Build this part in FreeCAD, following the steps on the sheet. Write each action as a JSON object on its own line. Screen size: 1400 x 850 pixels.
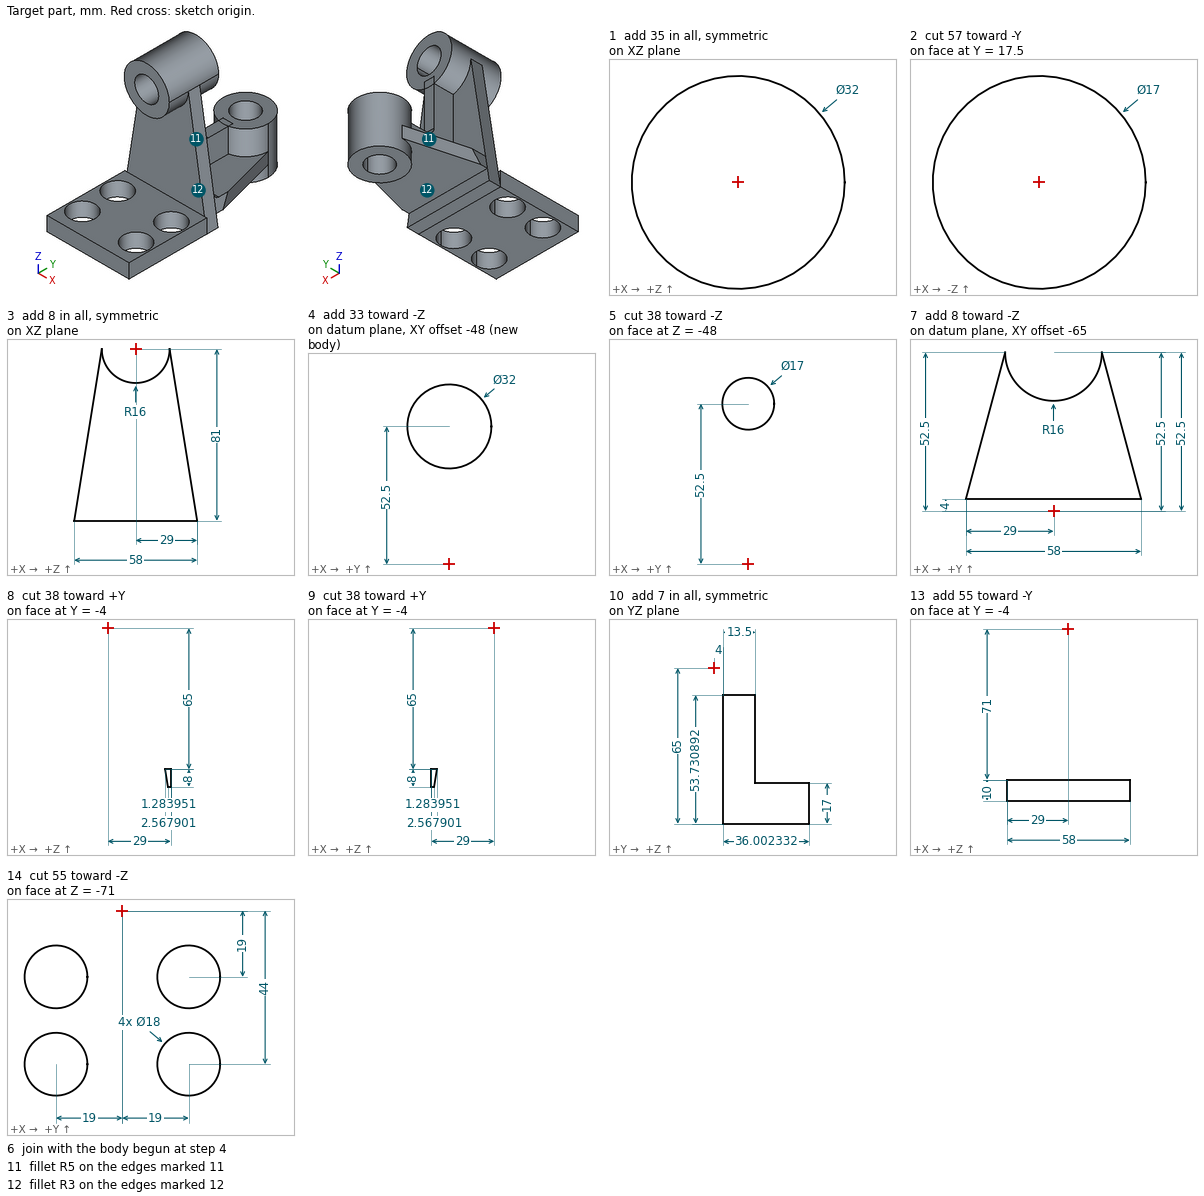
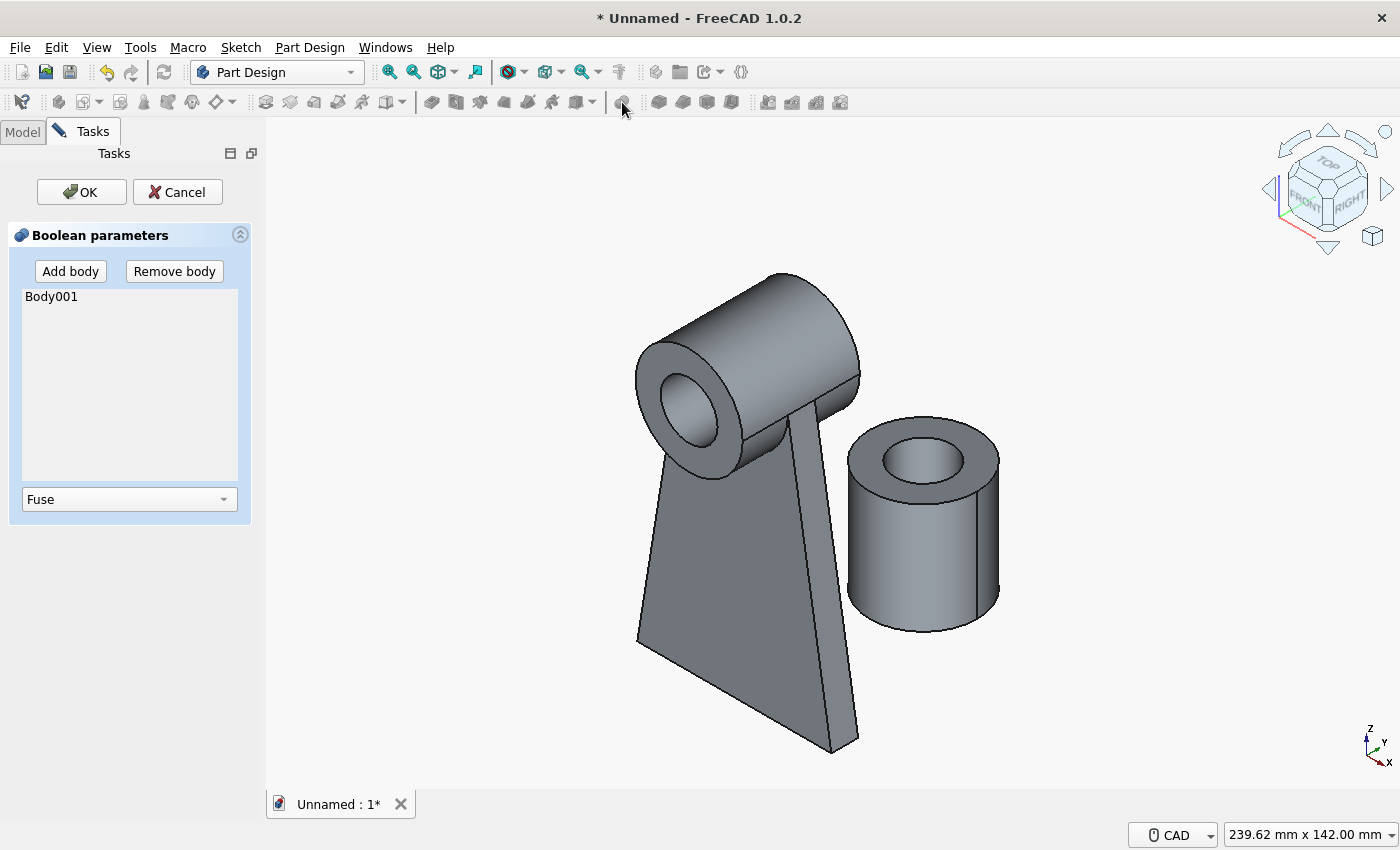
{"action": "left_click", "coordinate": [82, 192]}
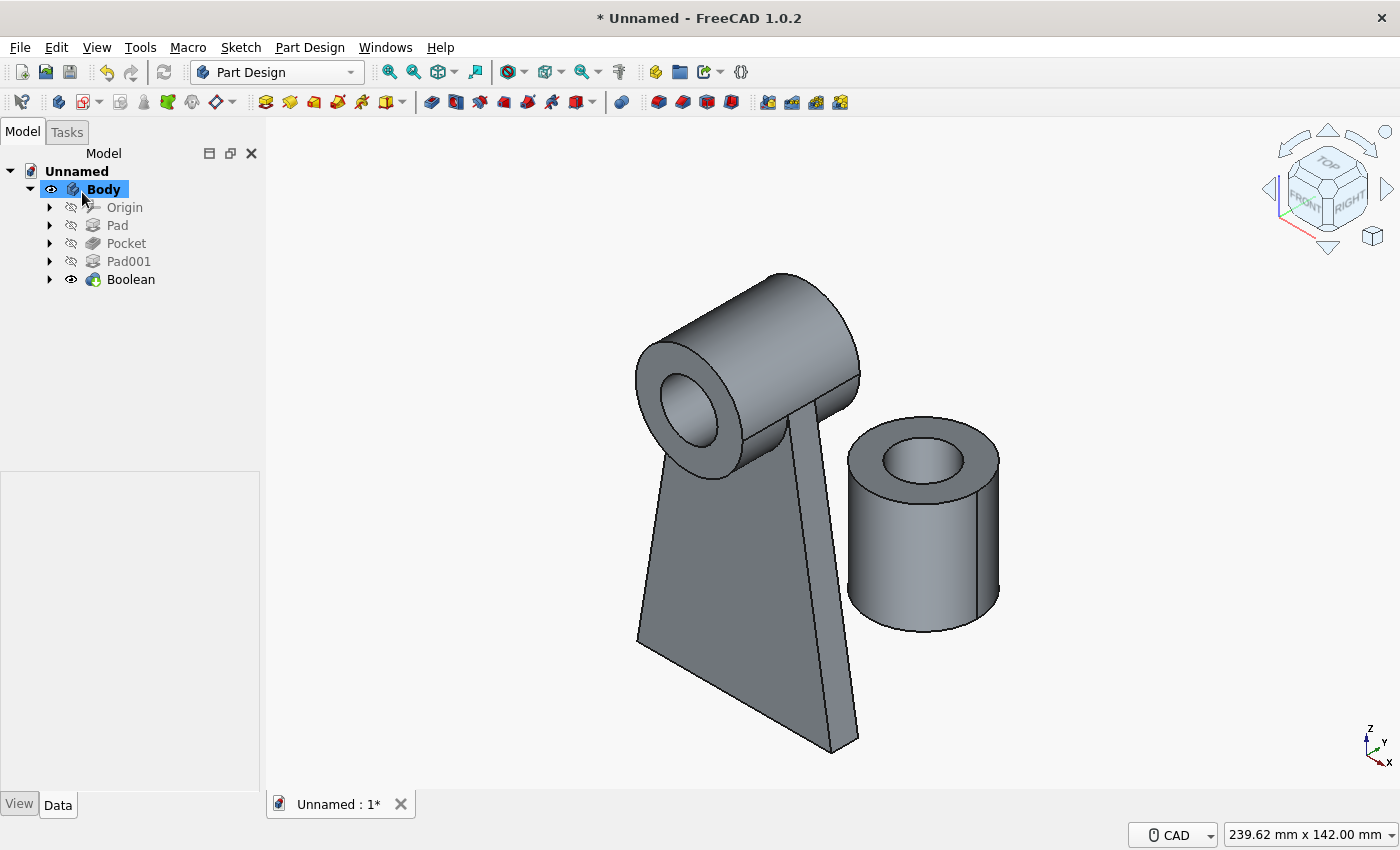
{"action": "left_click", "coordinate": [50, 207]}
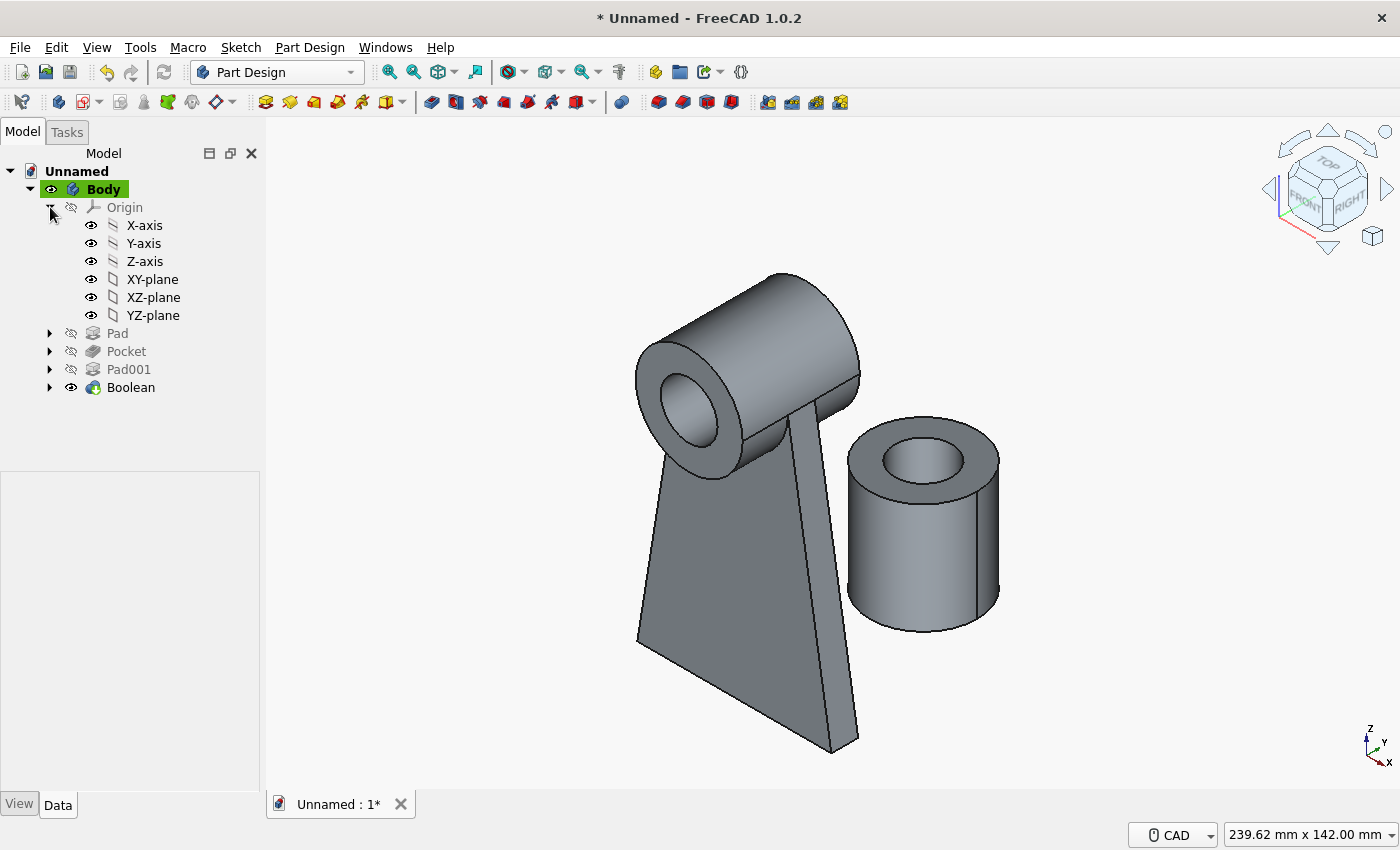
{"action": "left_click", "coordinate": [136, 279]}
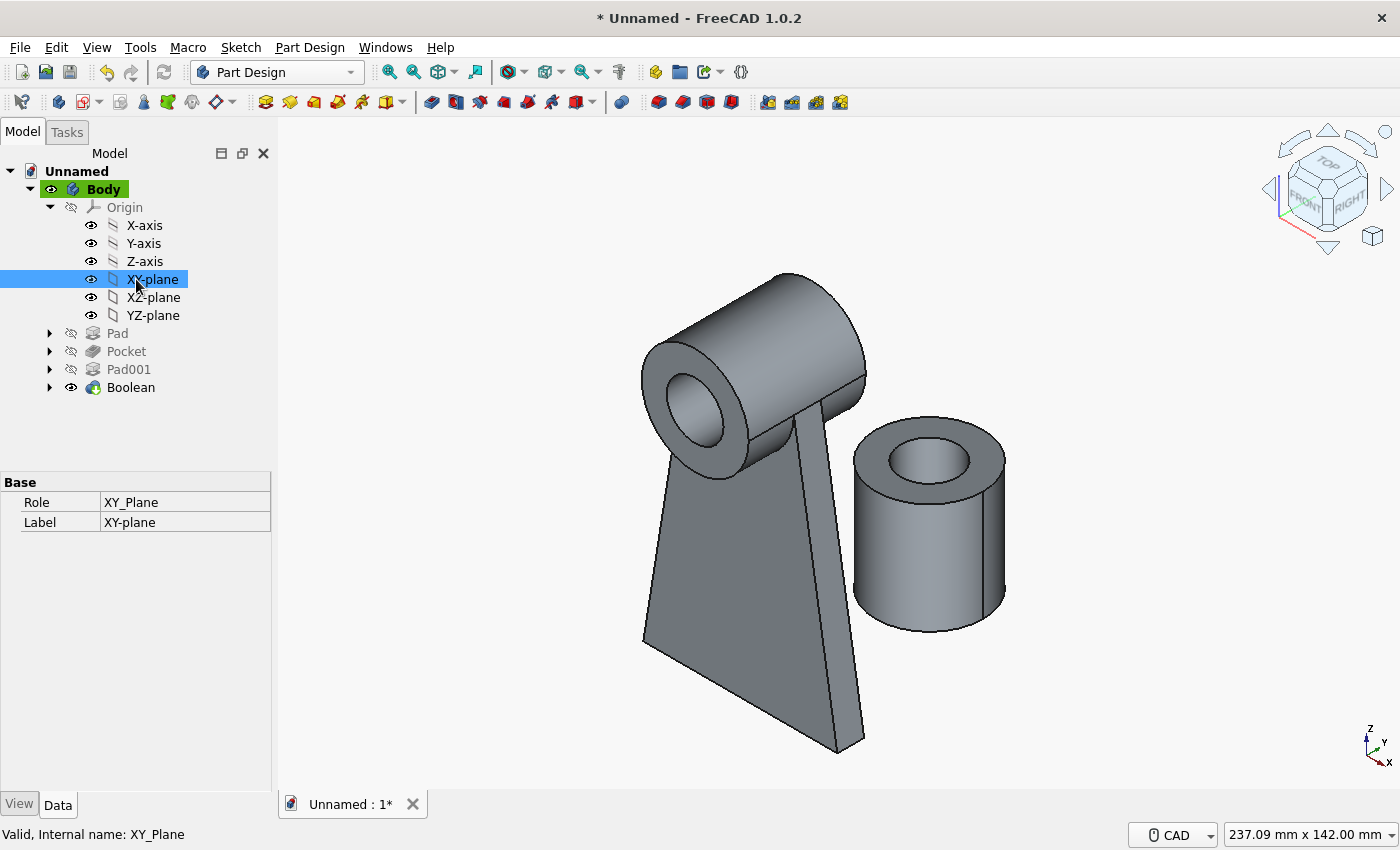
{"action": "left_click", "coordinate": [216, 102]}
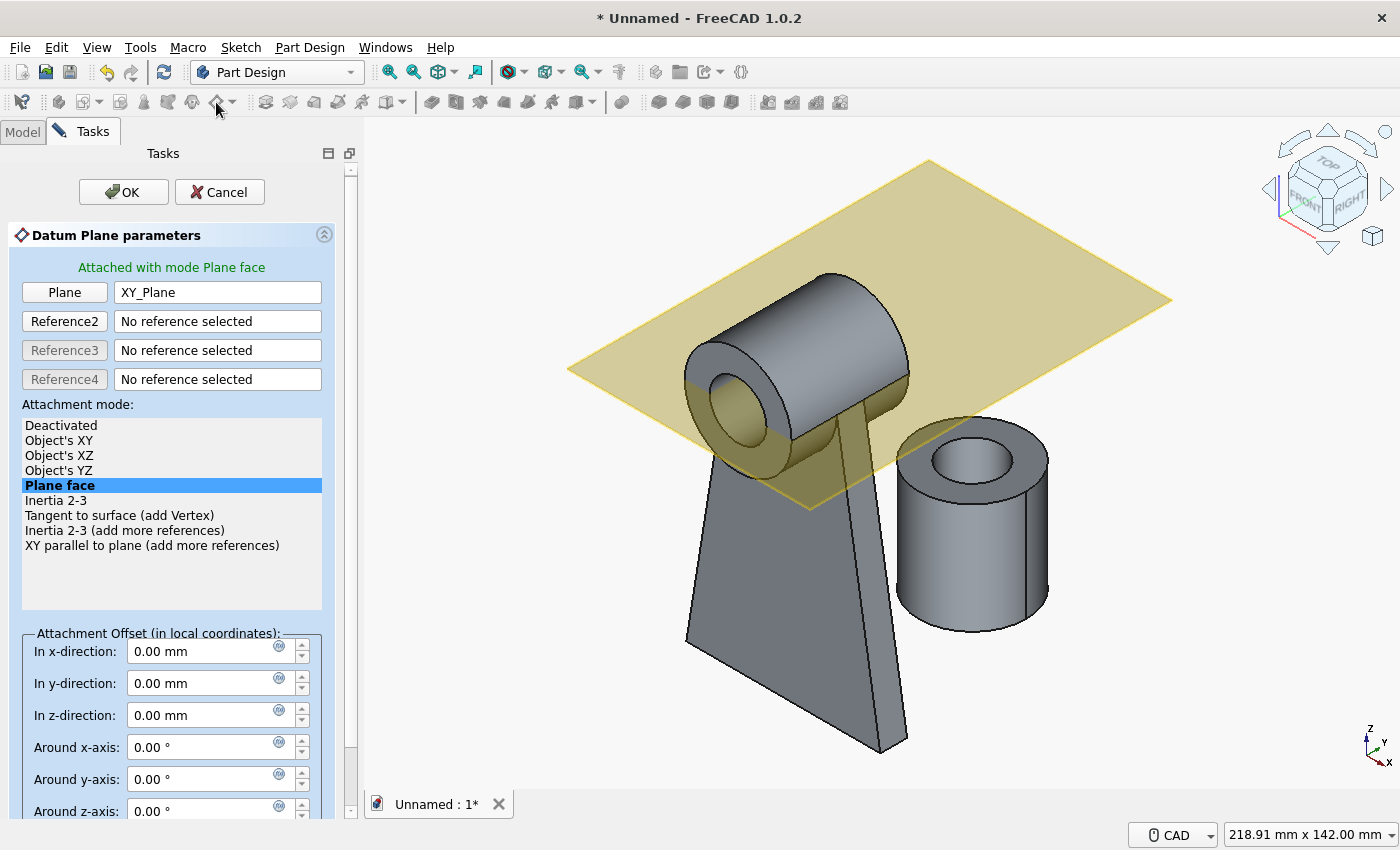
{"action": "triple_click", "coordinate": [210, 715]}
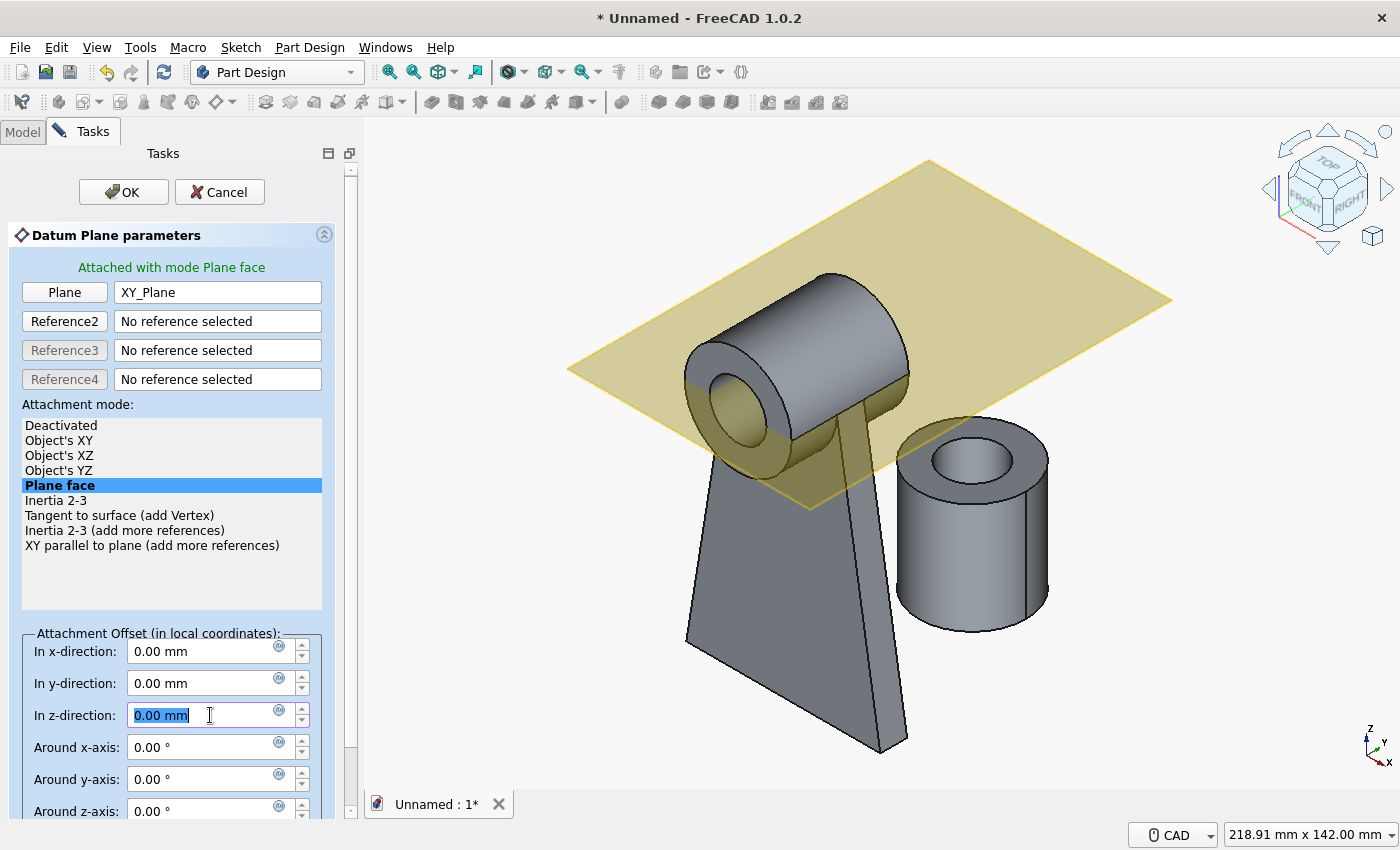
{"action": "type", "text": "-65"}
{"action": "key", "text": "Tab"}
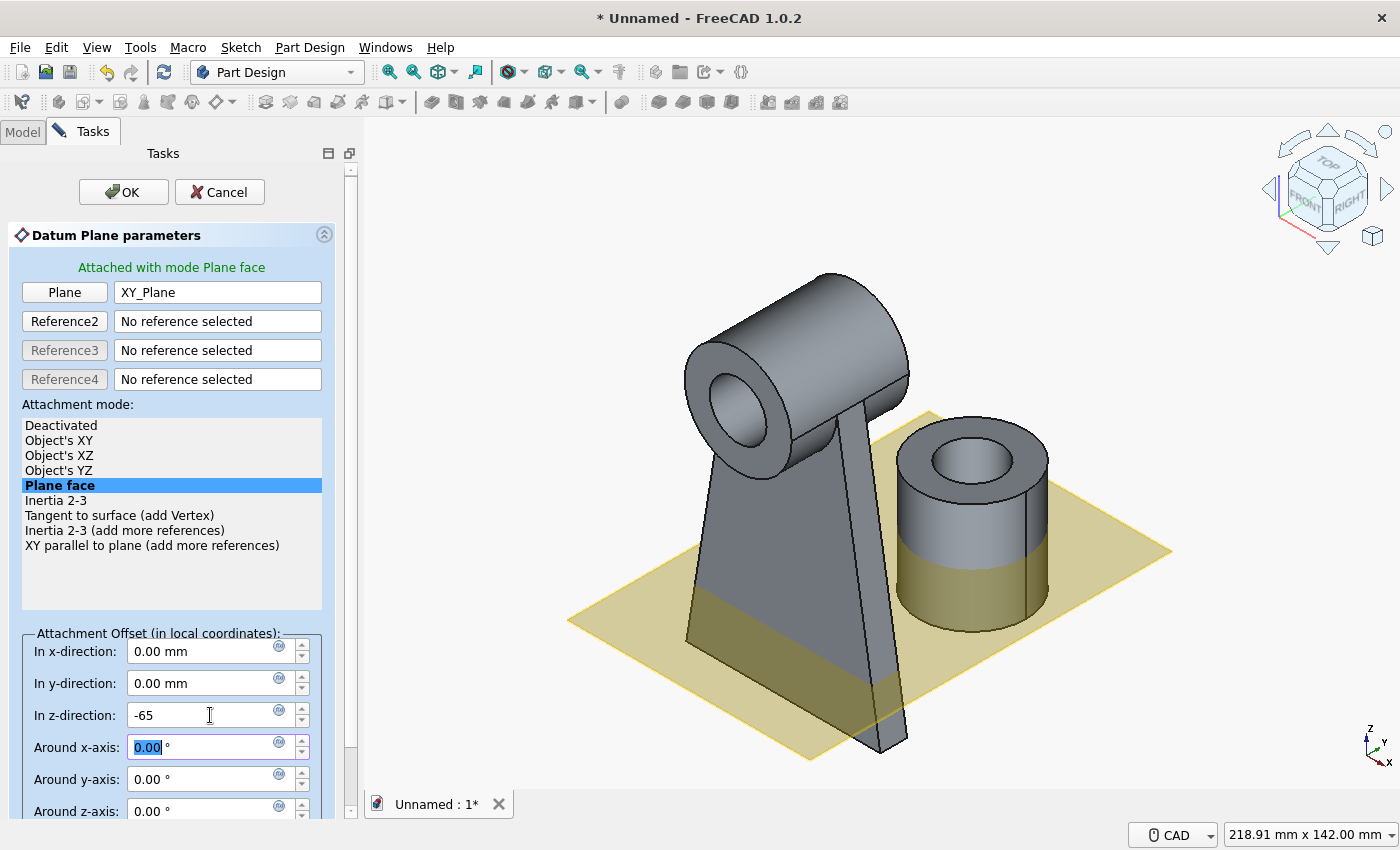
{"action": "left_click", "coordinate": [124, 192]}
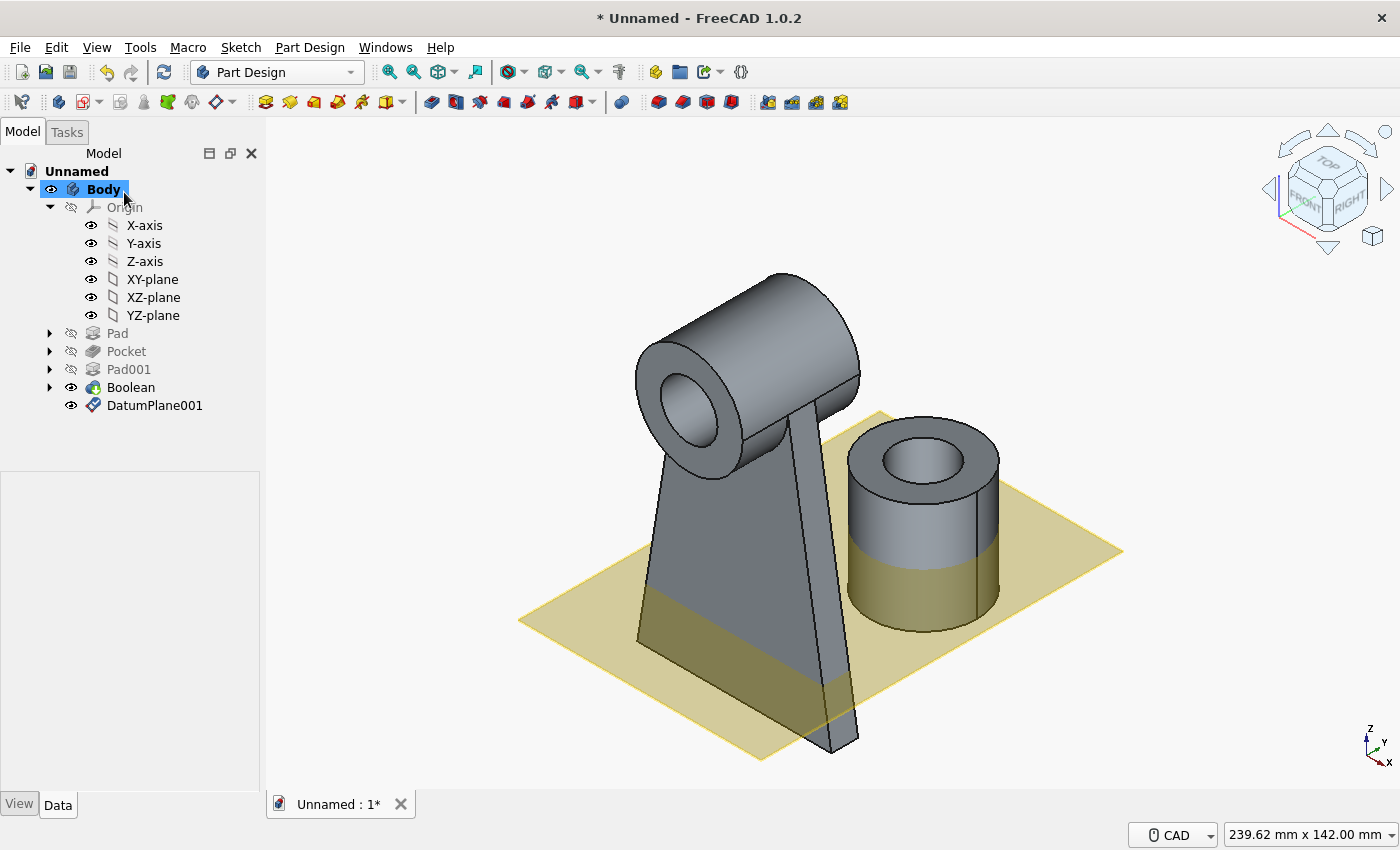
{"action": "left_click", "coordinate": [116, 405]}